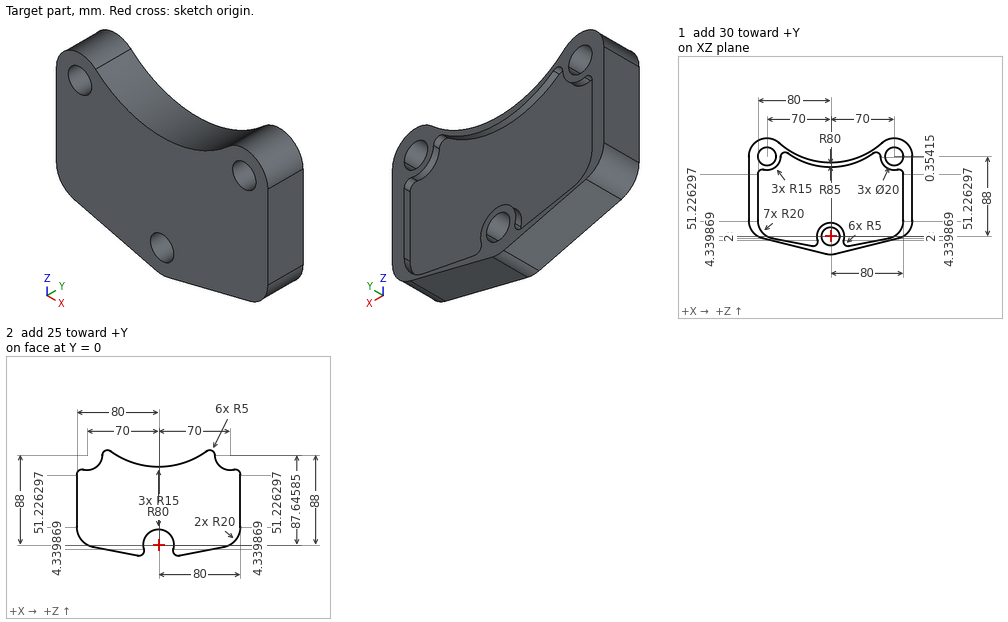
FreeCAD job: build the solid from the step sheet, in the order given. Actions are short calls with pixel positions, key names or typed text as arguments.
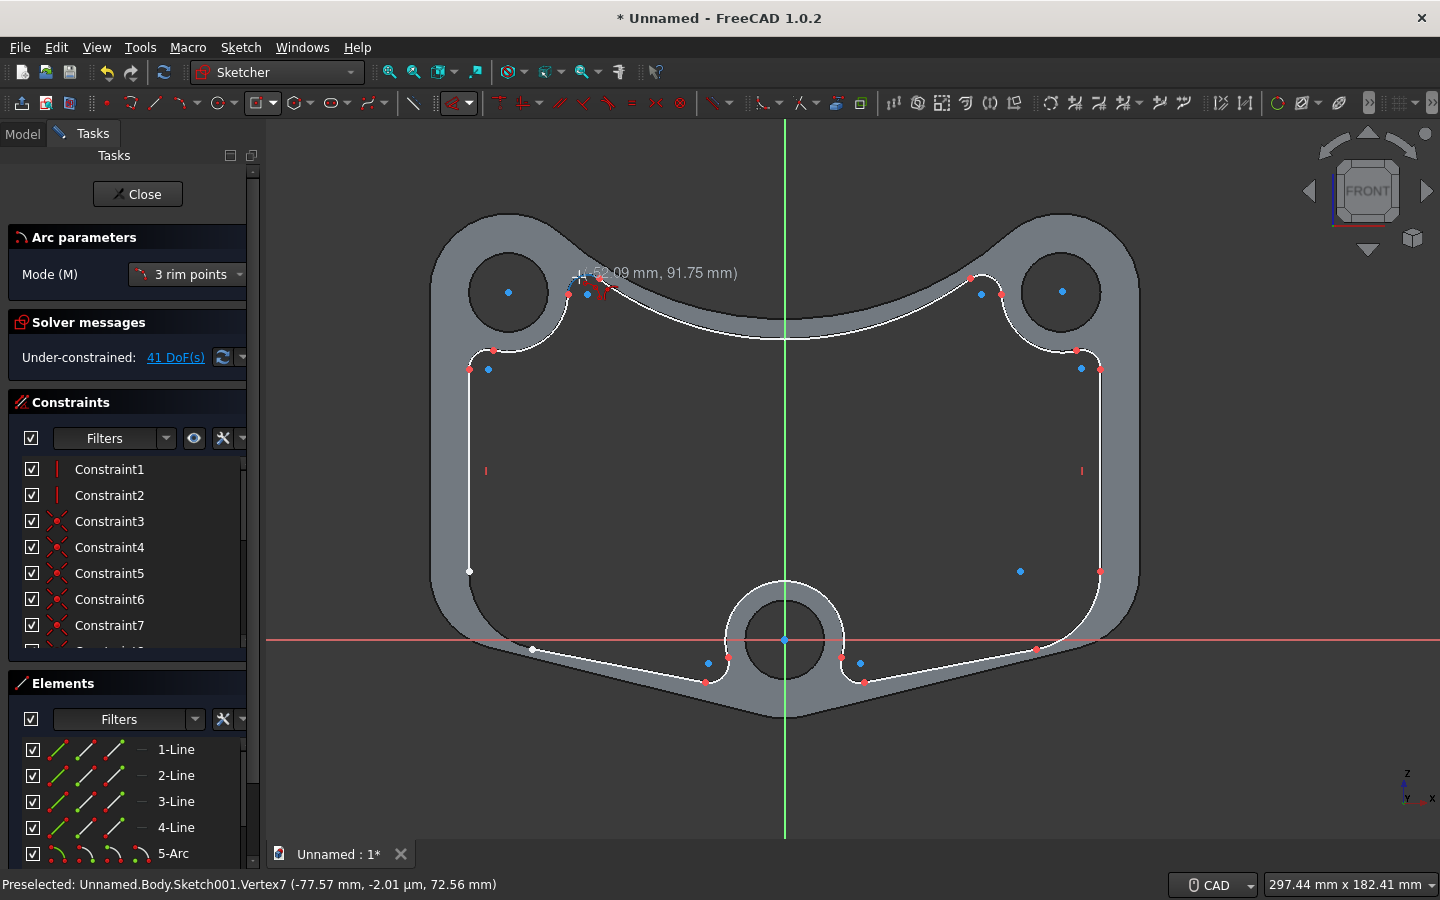
click(469, 572)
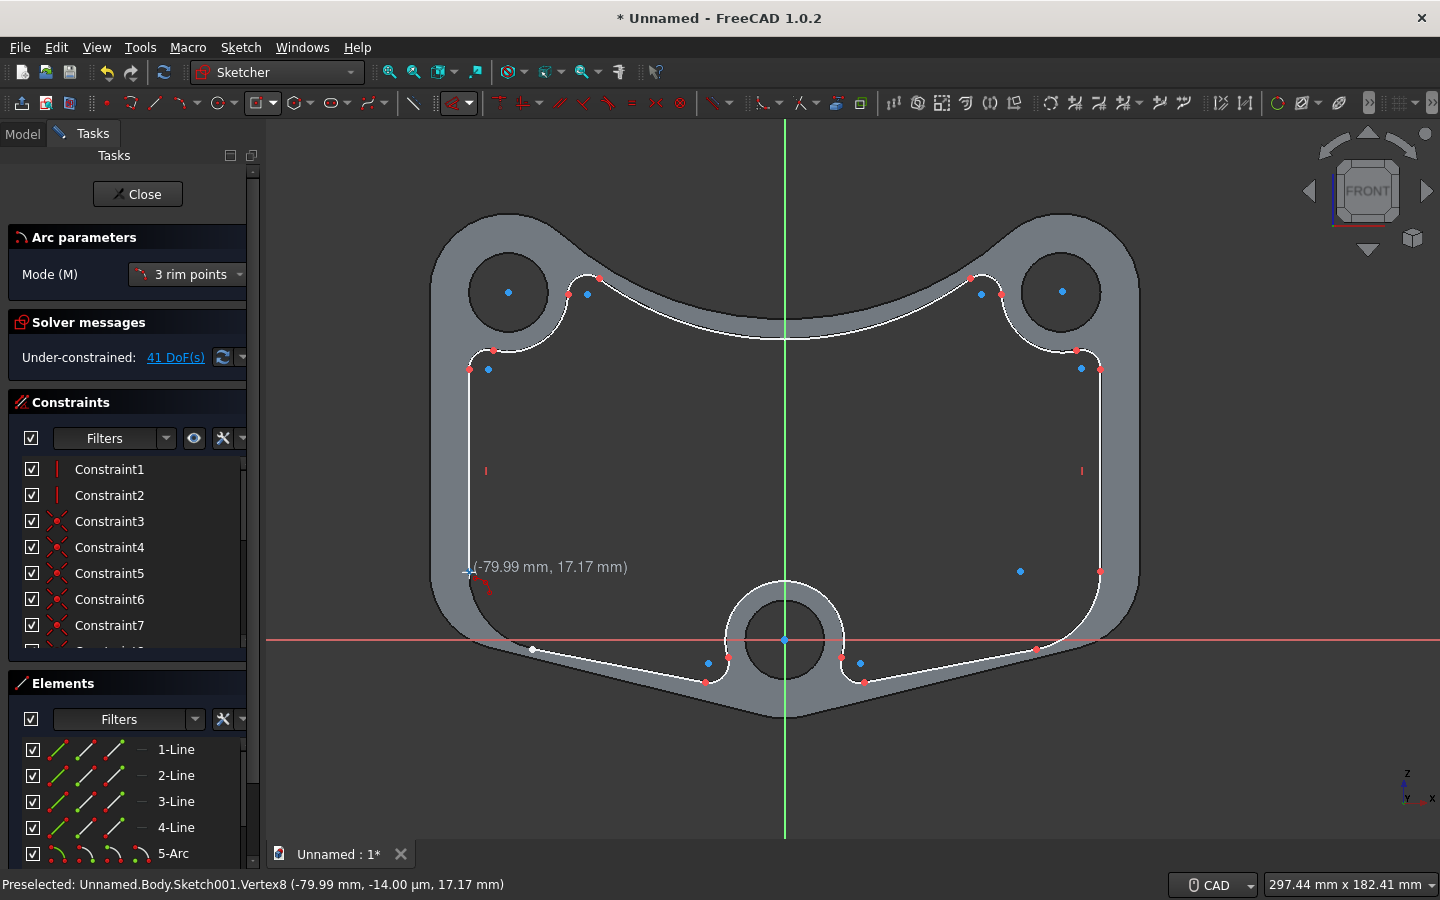
scroll(533, 649, up, 3)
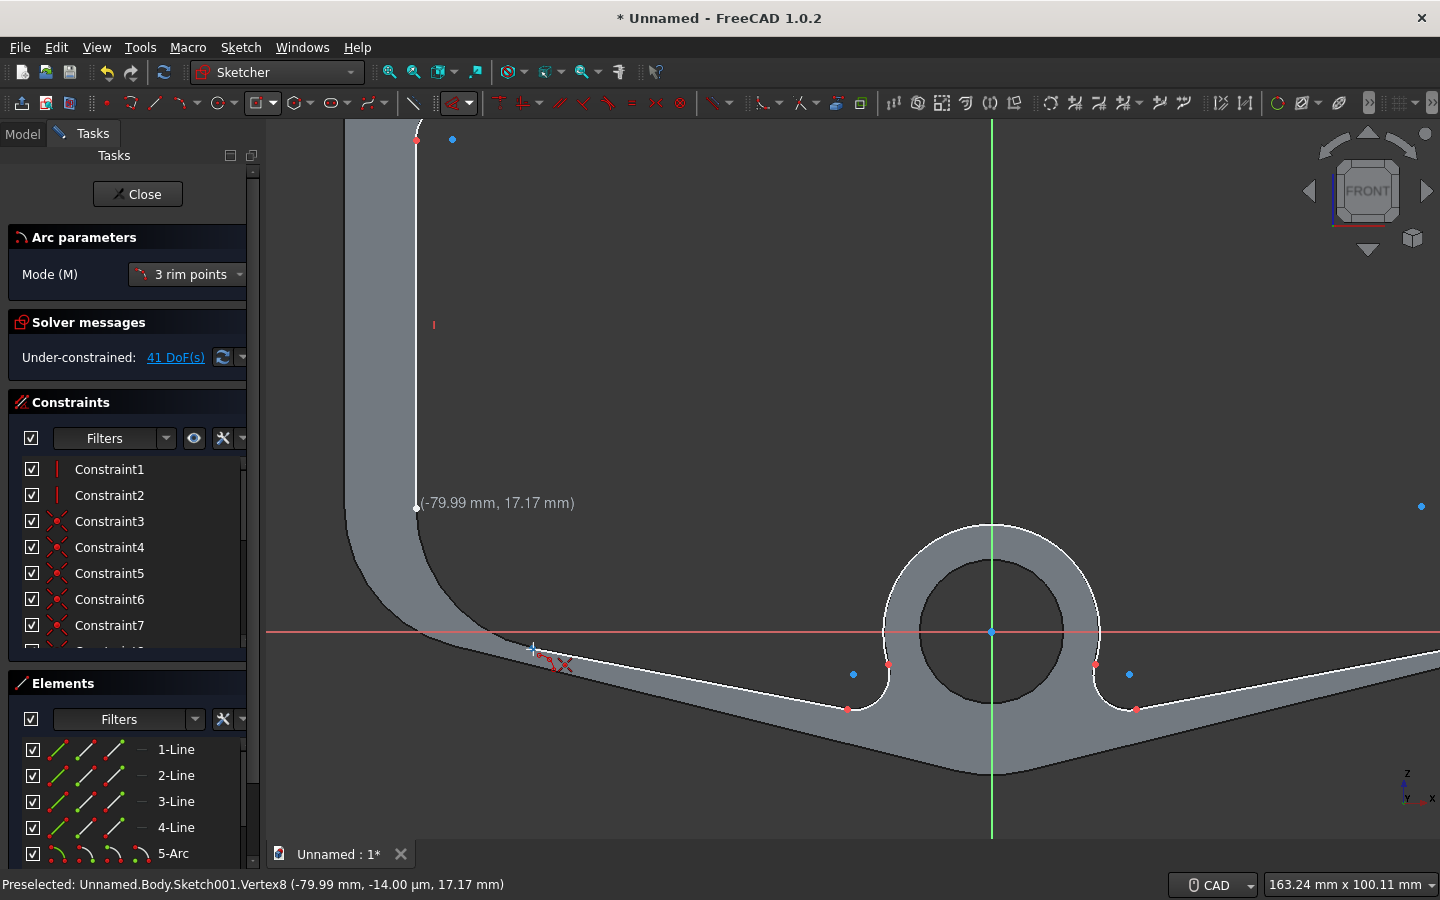
click(532, 649)
click(449, 598)
key(Escape)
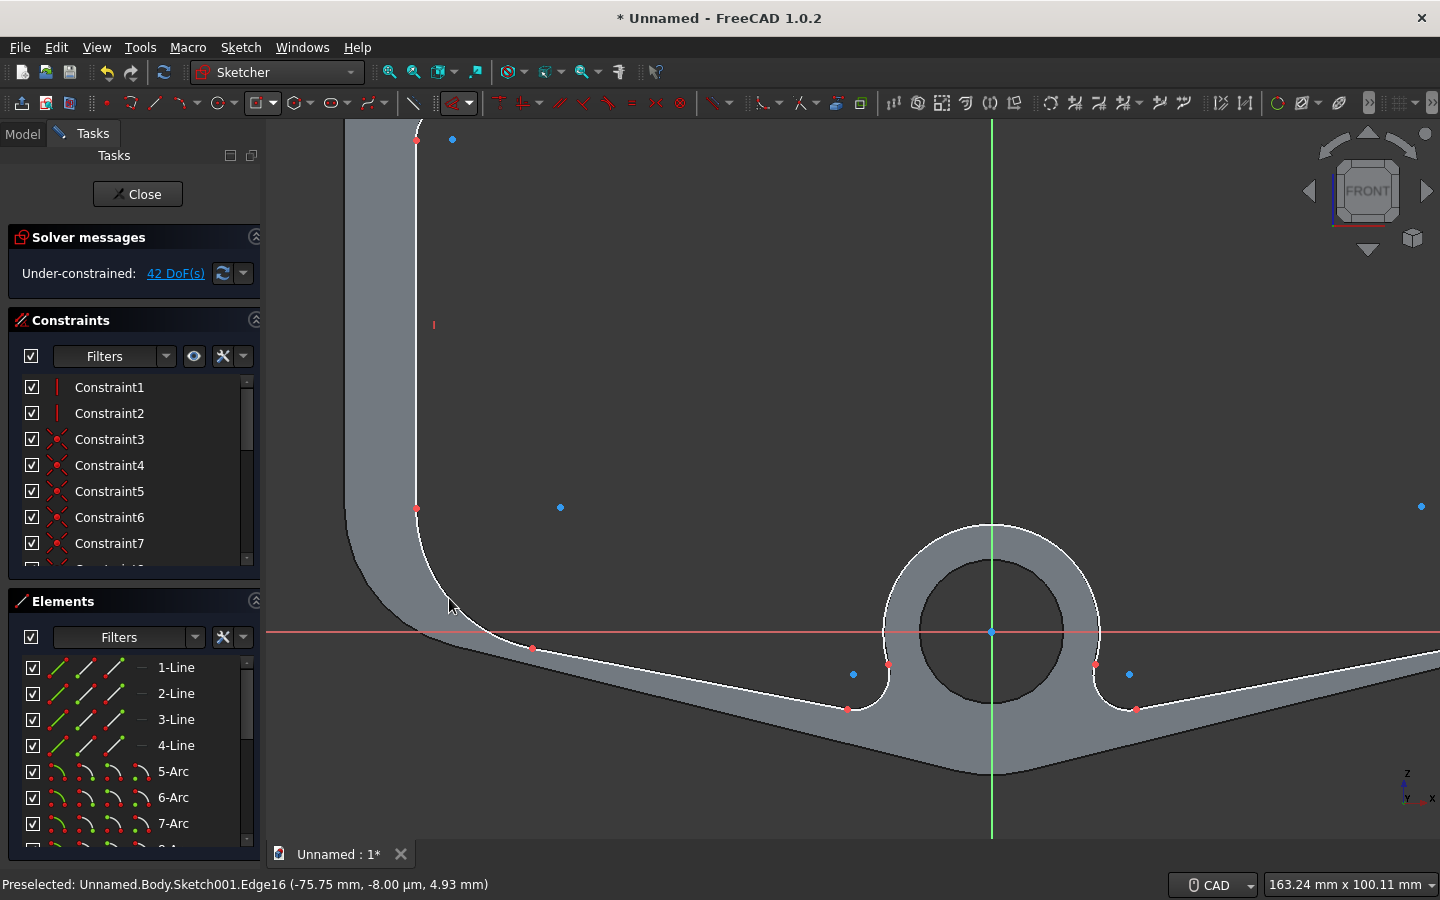
click(627, 667)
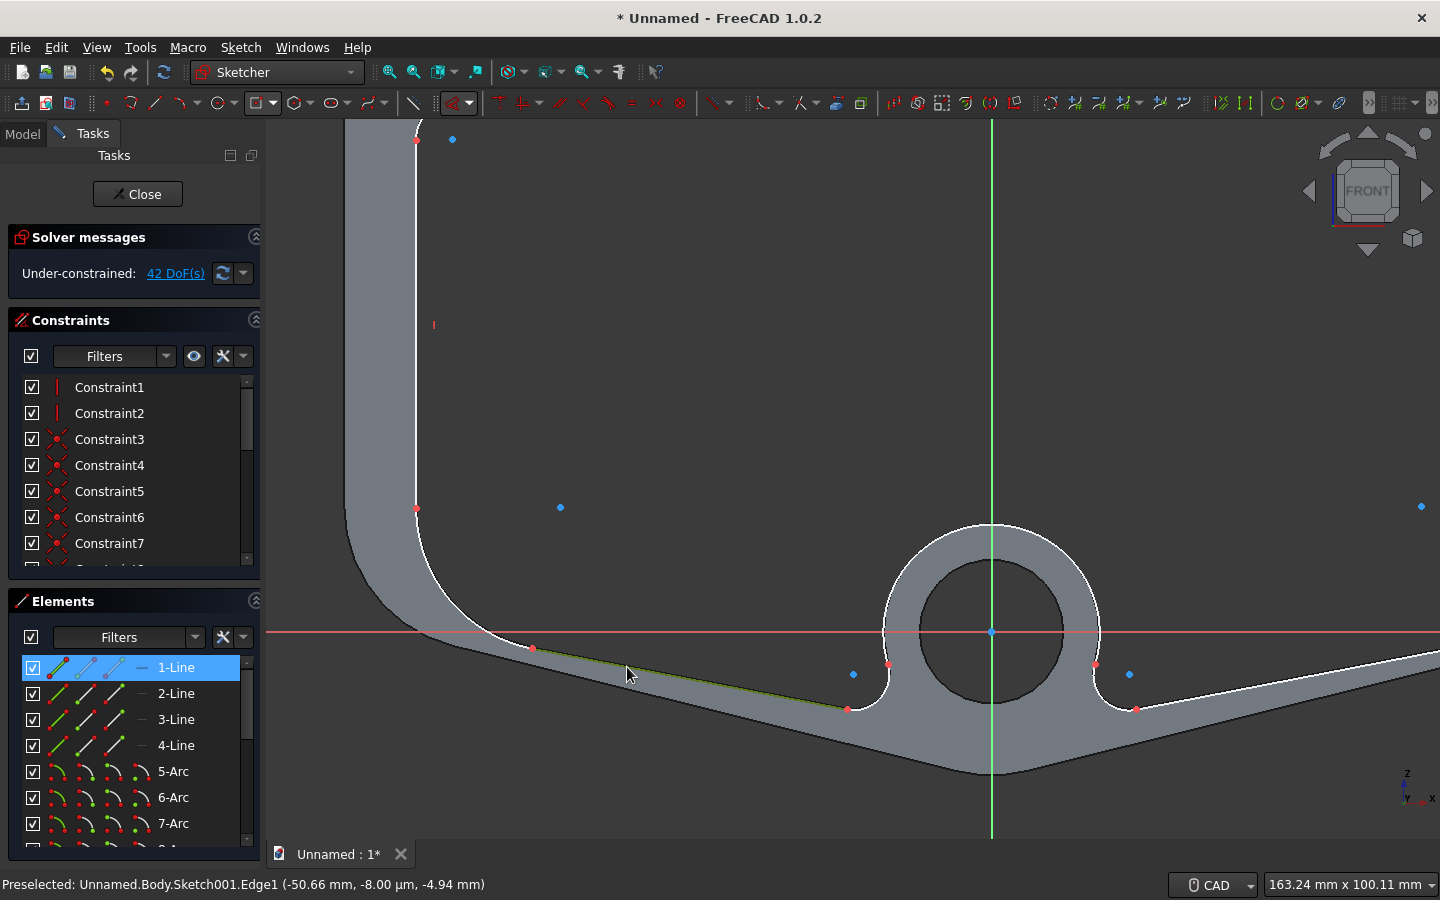
click(869, 707)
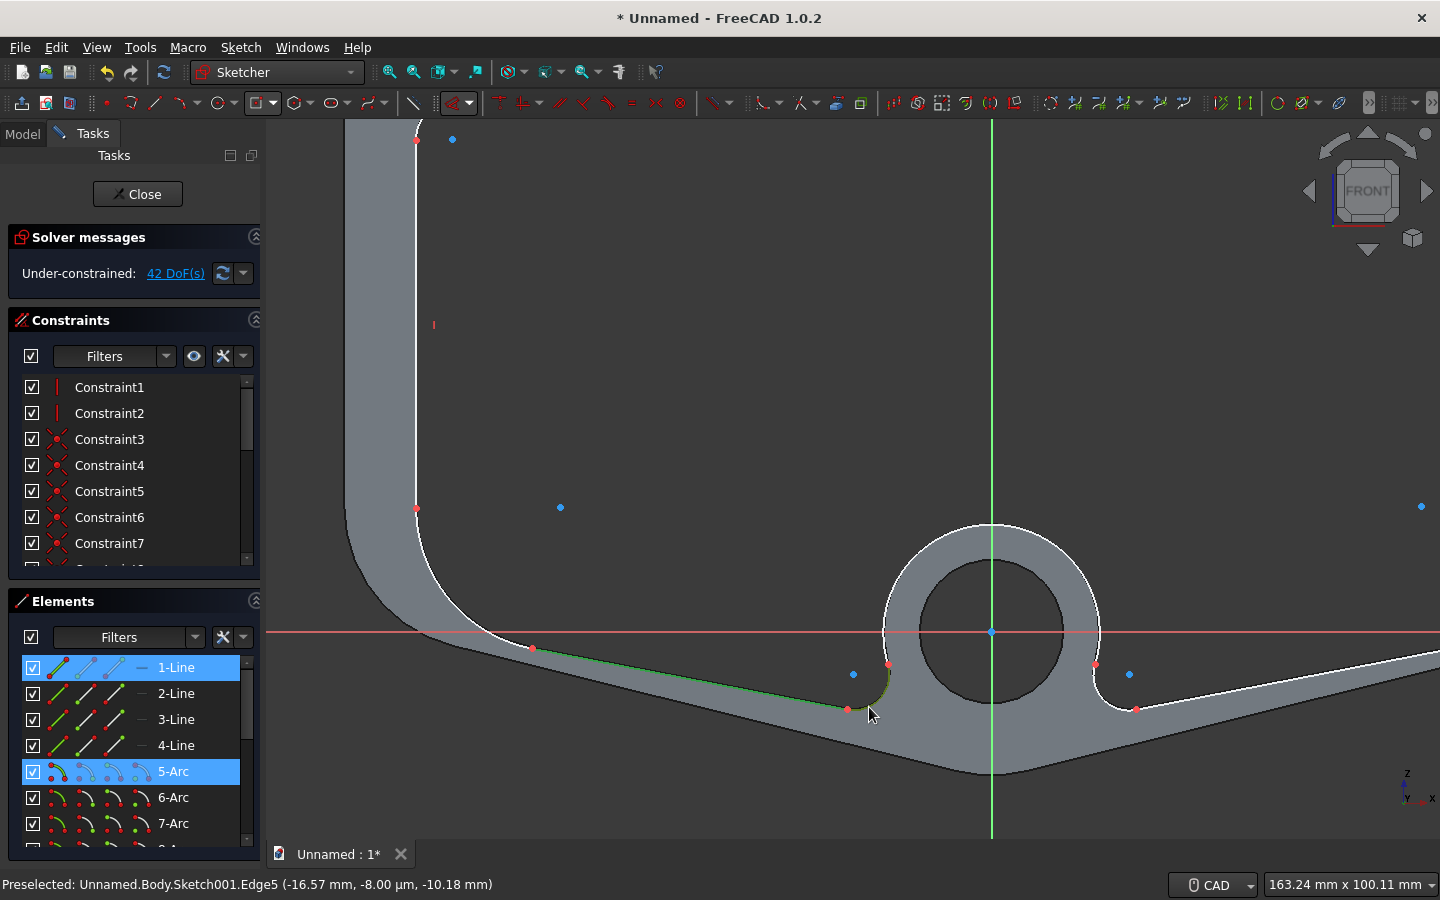
key(t)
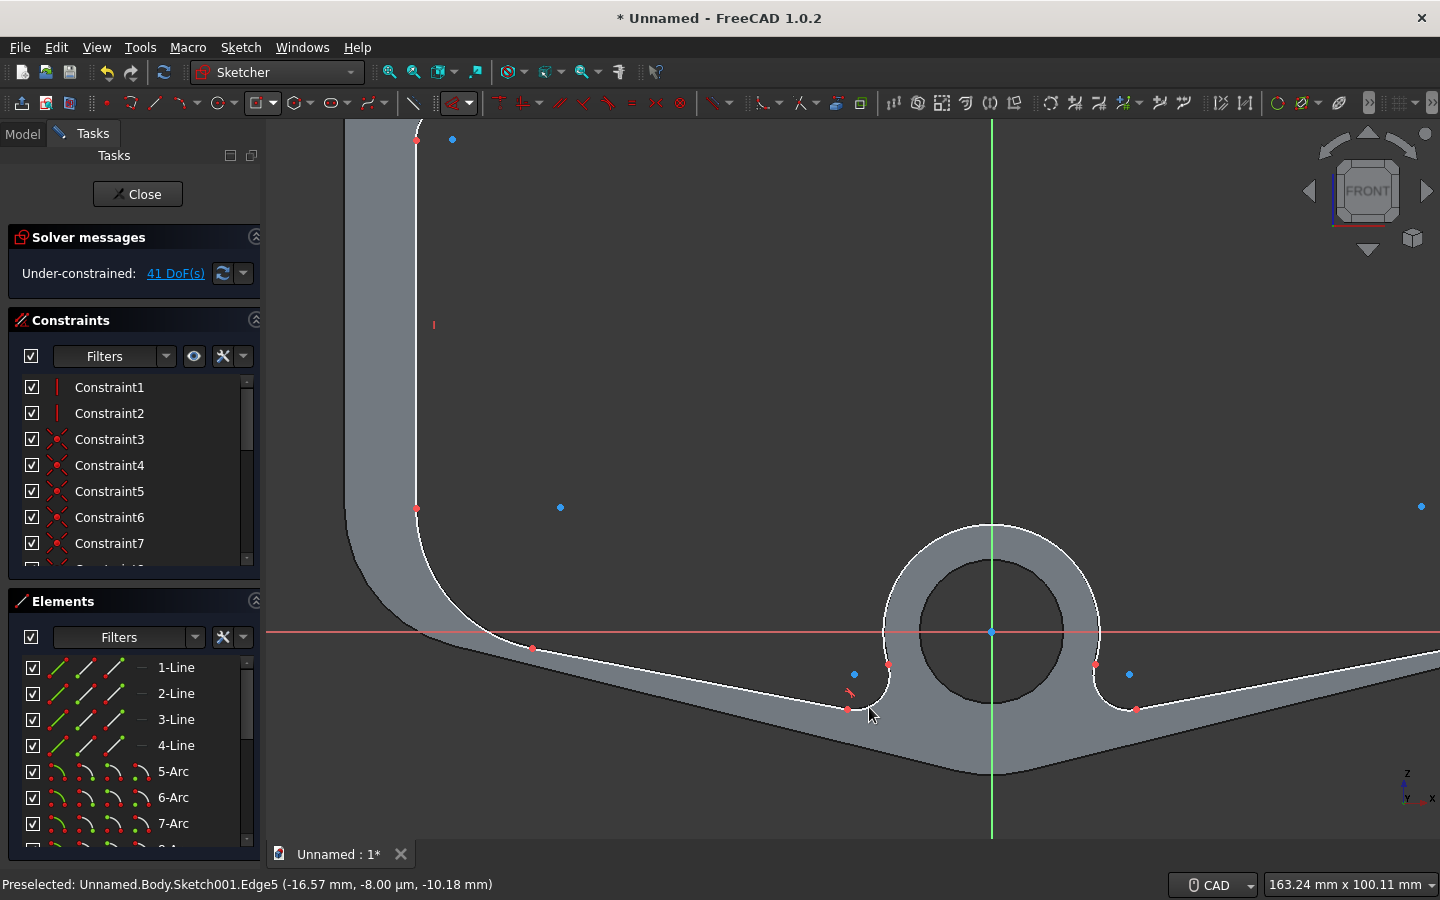
click(627, 667)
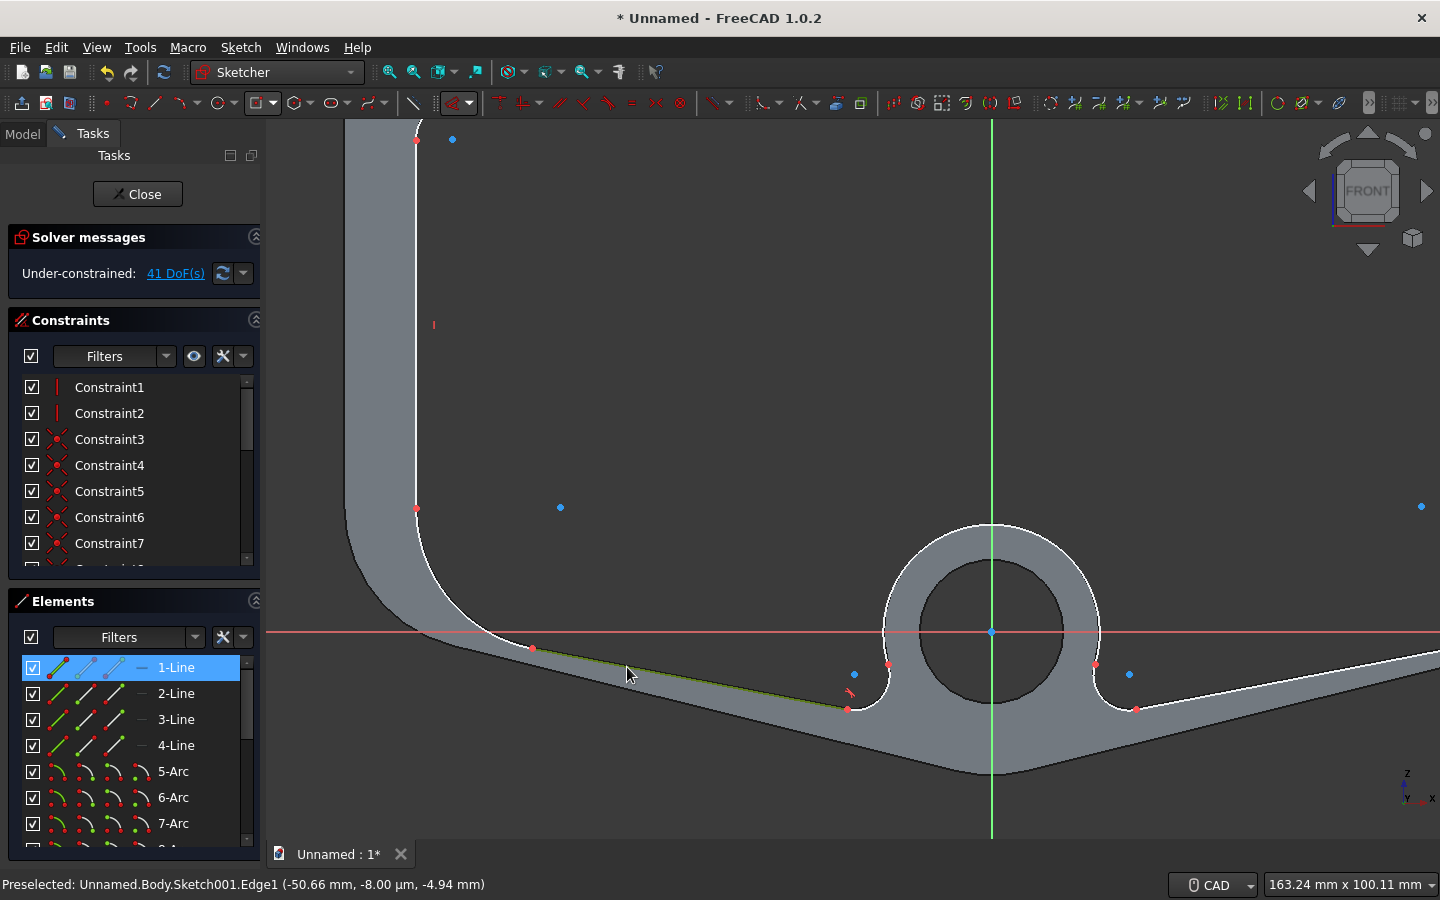
click(428, 566)